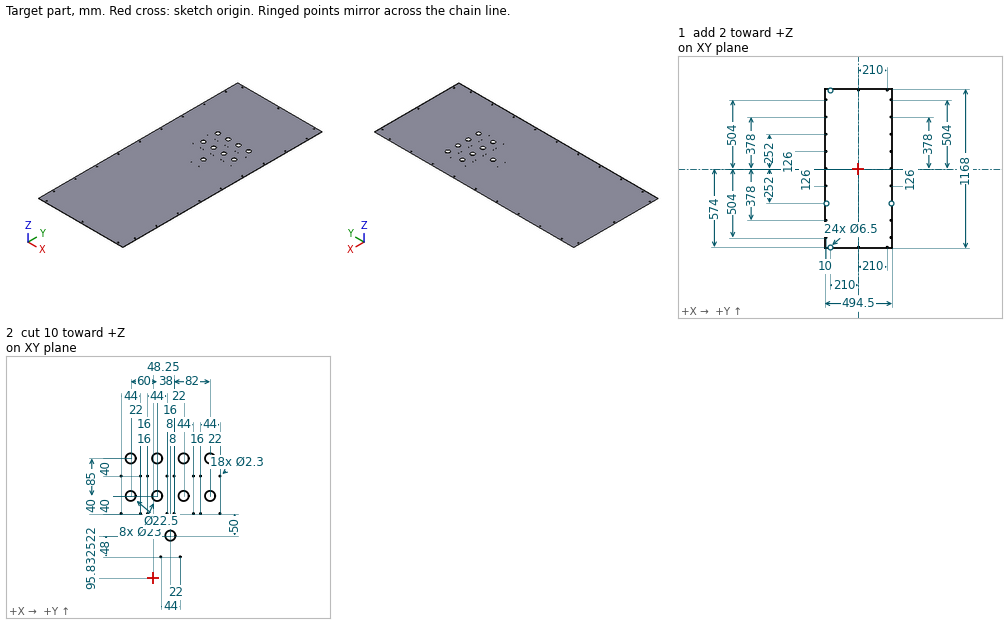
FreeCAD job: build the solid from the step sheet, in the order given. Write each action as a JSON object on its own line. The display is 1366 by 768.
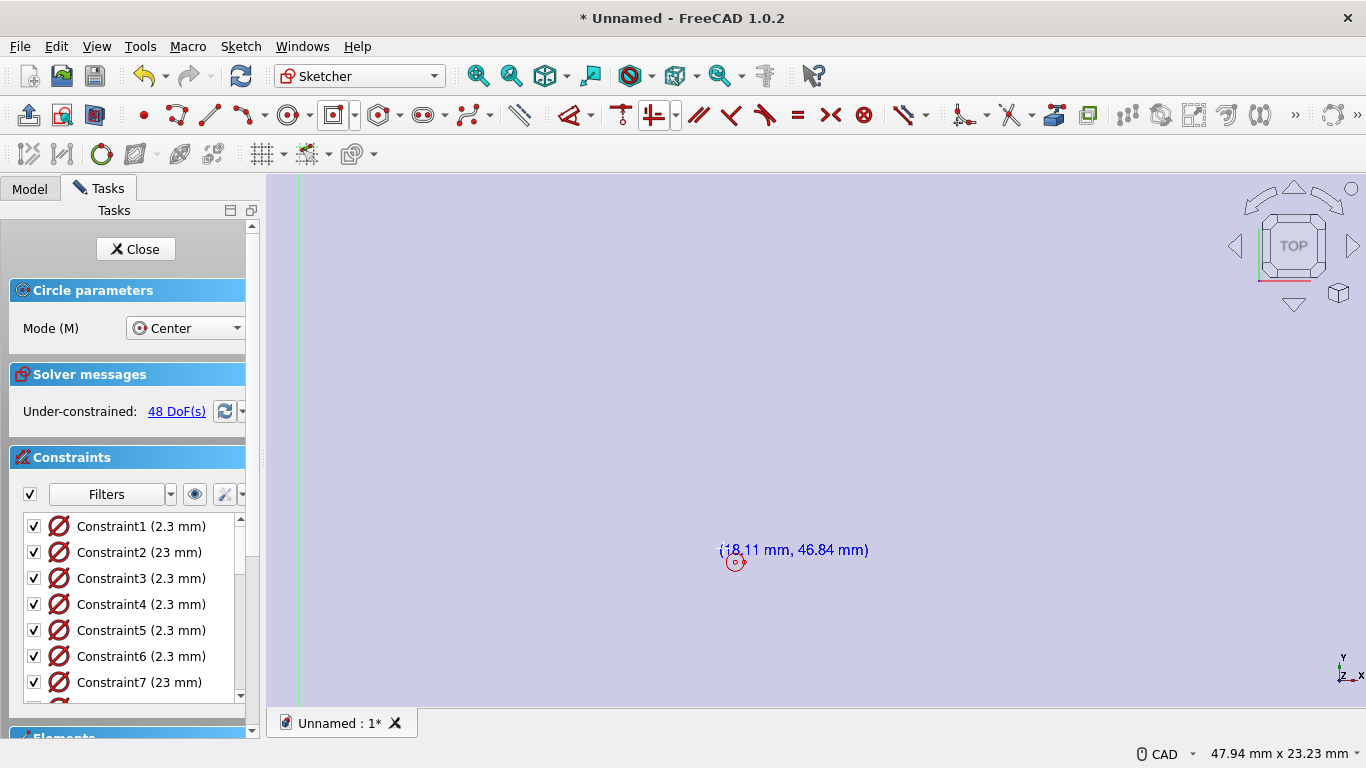
{"action": "scroll", "coordinate": [723, 548], "scroll_direction": "down", "scroll_amount": 15}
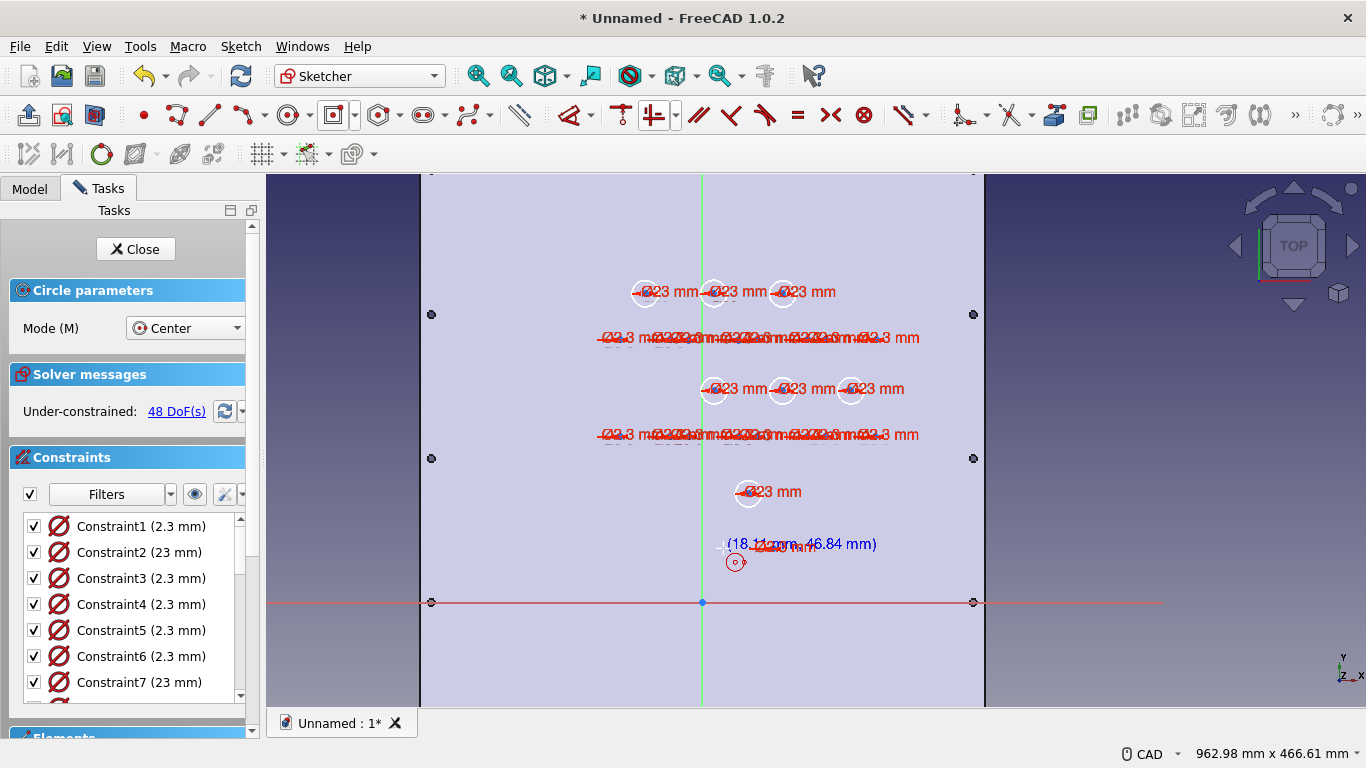
{"action": "left_click", "coordinate": [723, 548]}
{"action": "mouse_move", "coordinate": [724, 547]}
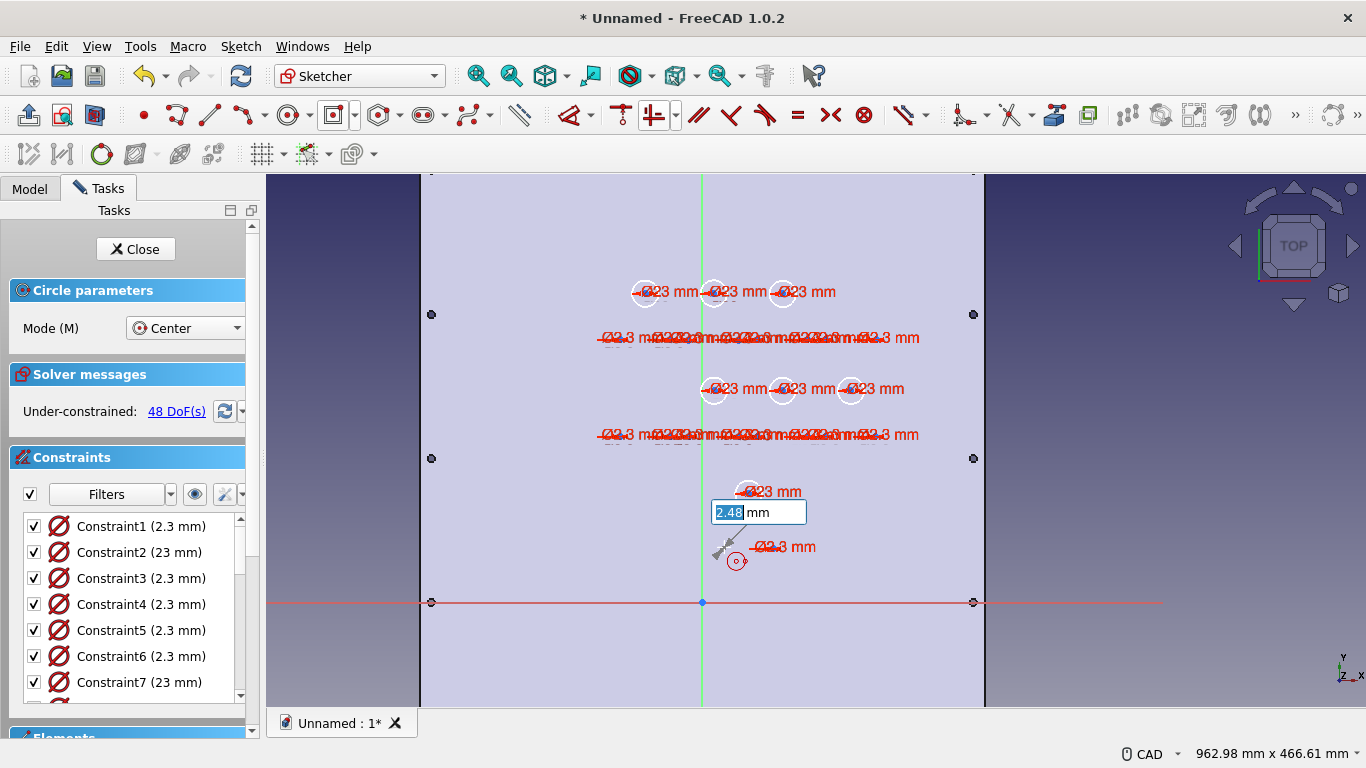
{"action": "type", "text": "2.3"}
{"action": "key", "text": "Return"}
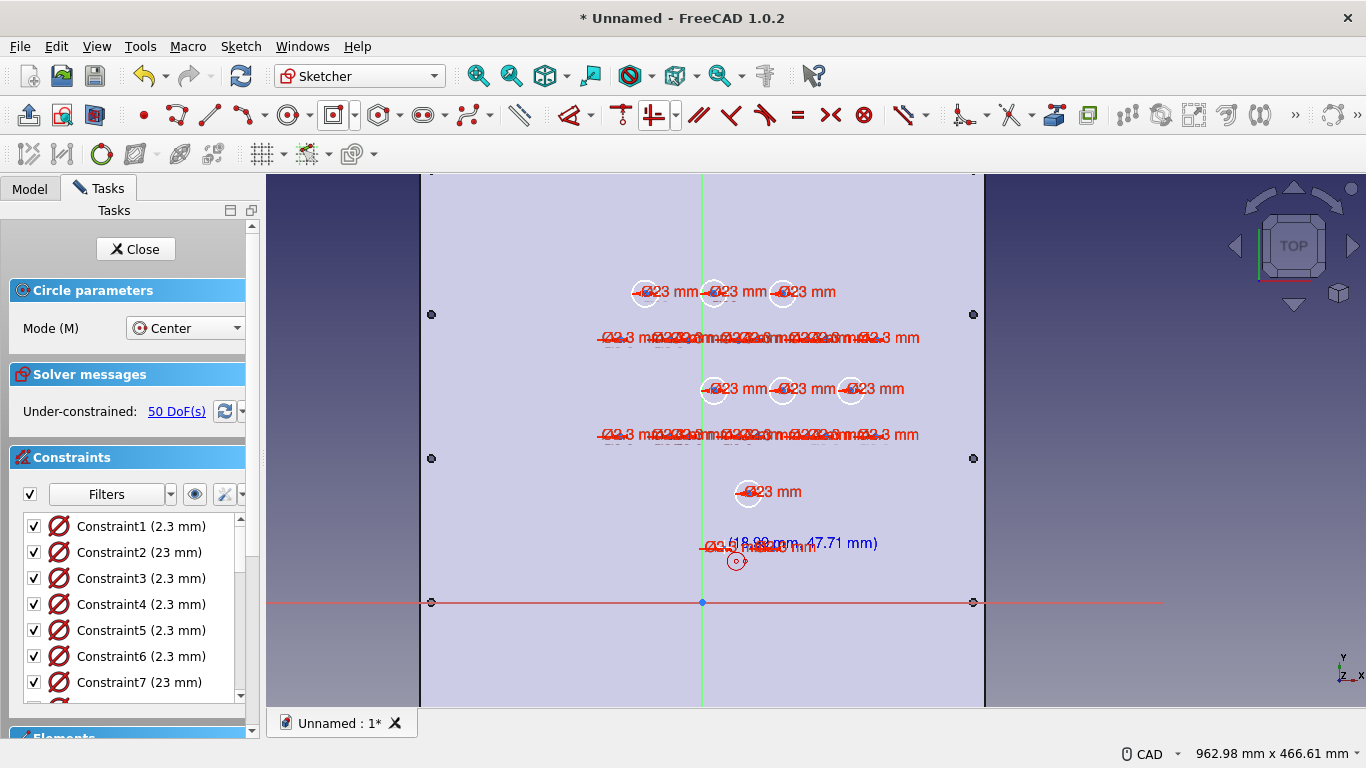
{"action": "scroll", "coordinate": [851, 293], "scroll_direction": "up", "scroll_amount": 3}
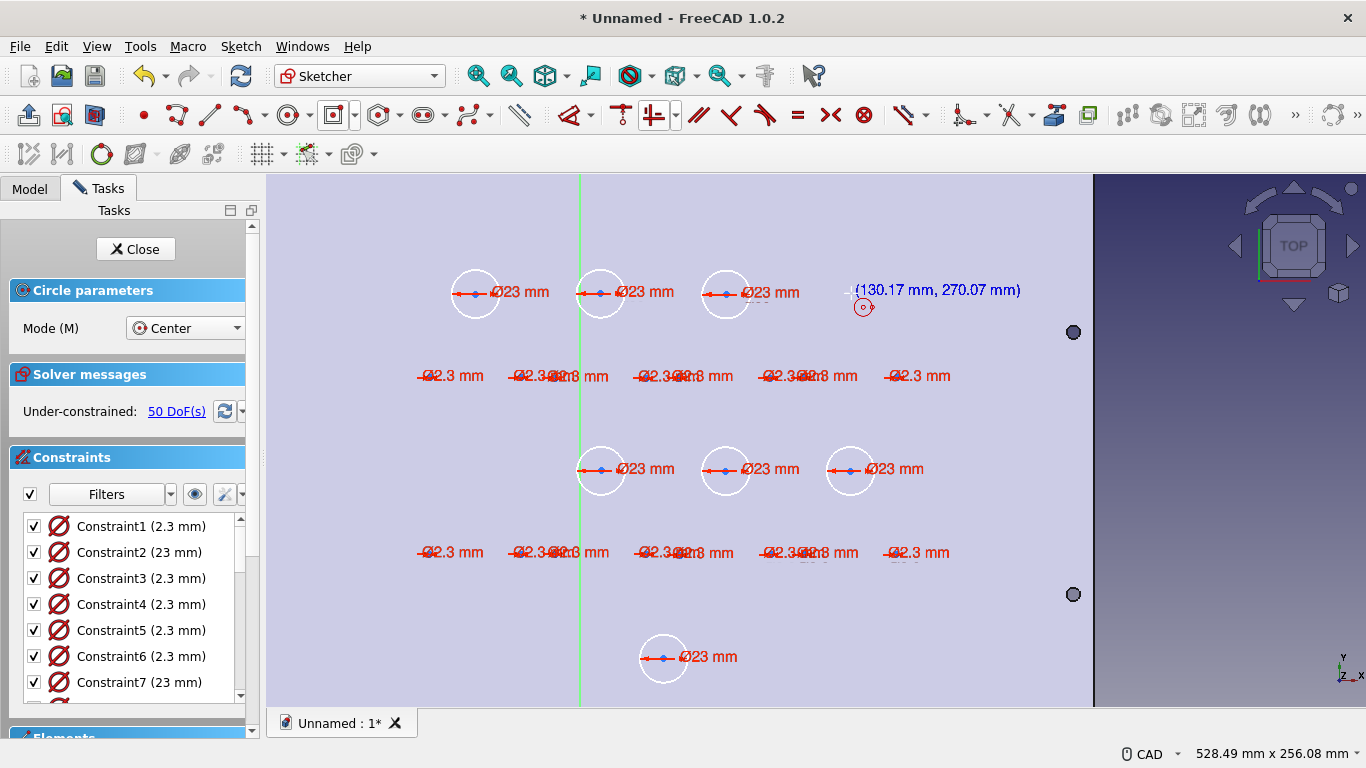
{"action": "left_click", "coordinate": [851, 293]}
{"action": "mouse_move", "coordinate": [868, 276]}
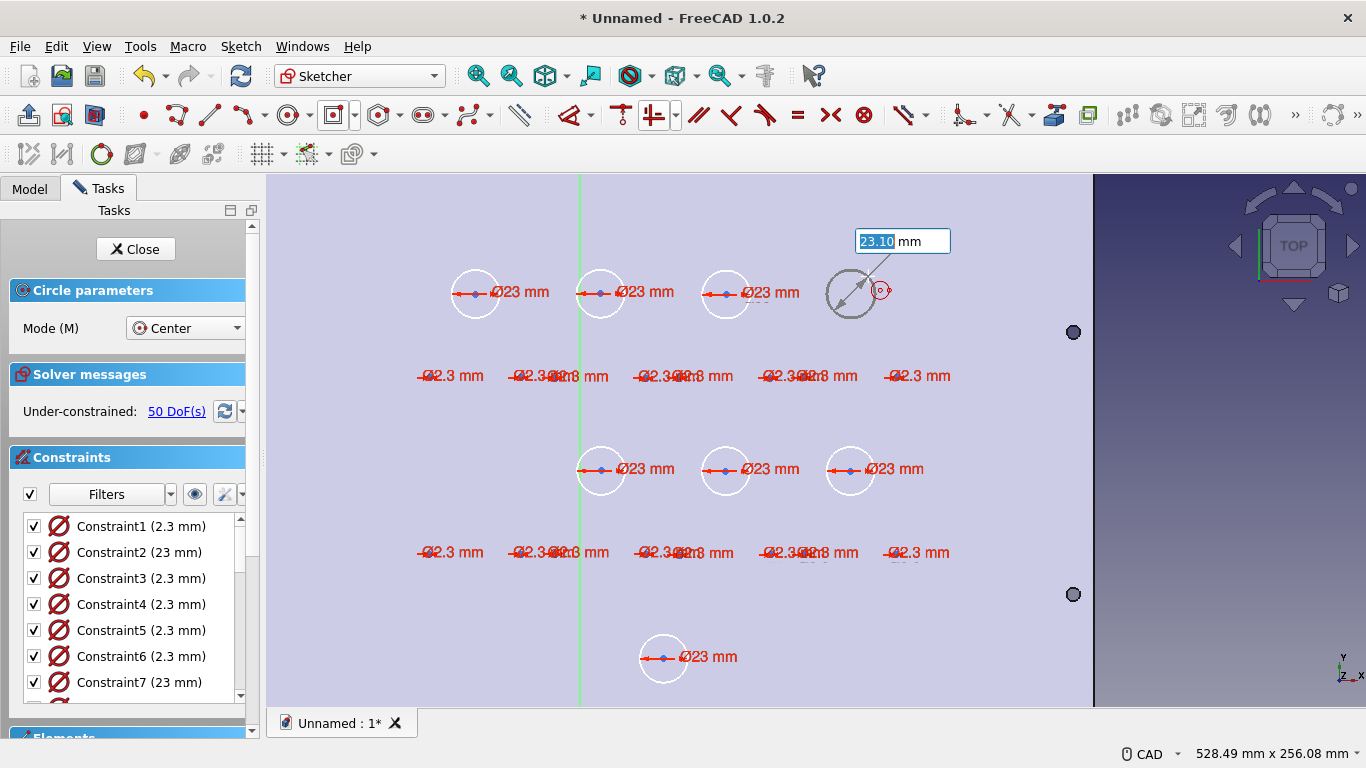
{"action": "type", "text": "23"}
{"action": "key", "text": "Return"}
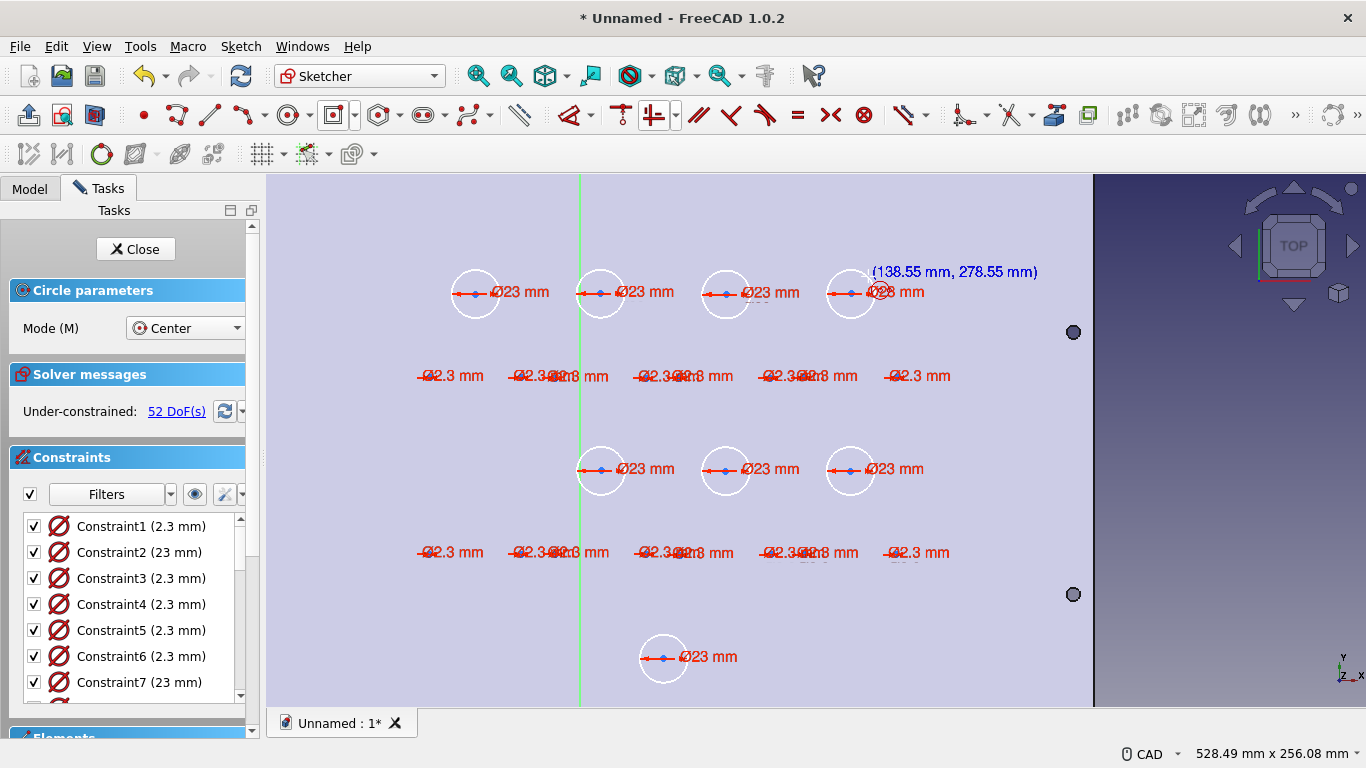
{"action": "left_click", "coordinate": [476, 470]}
{"action": "mouse_move", "coordinate": [493, 453]}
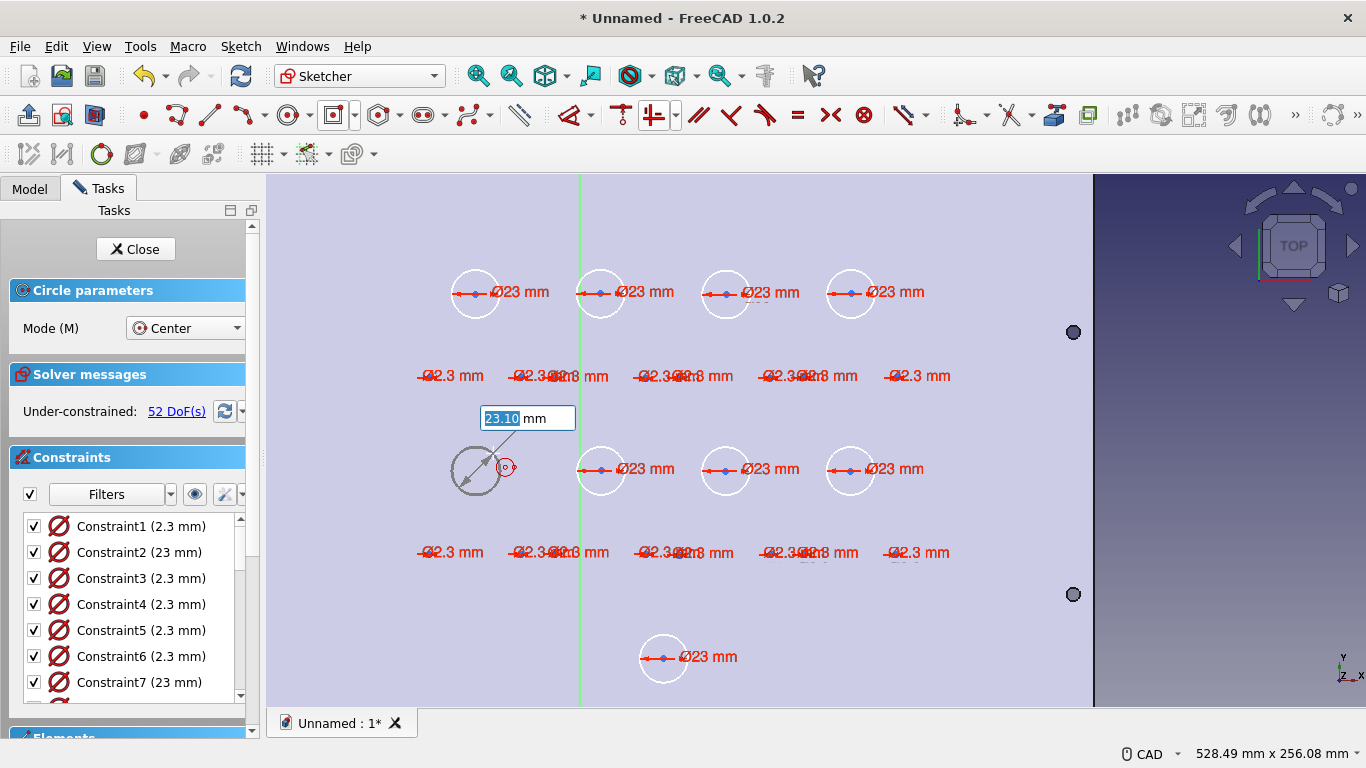
{"action": "type", "text": "22.5"}
{"action": "key", "text": "Return"}
{"action": "key", "text": "Escape"}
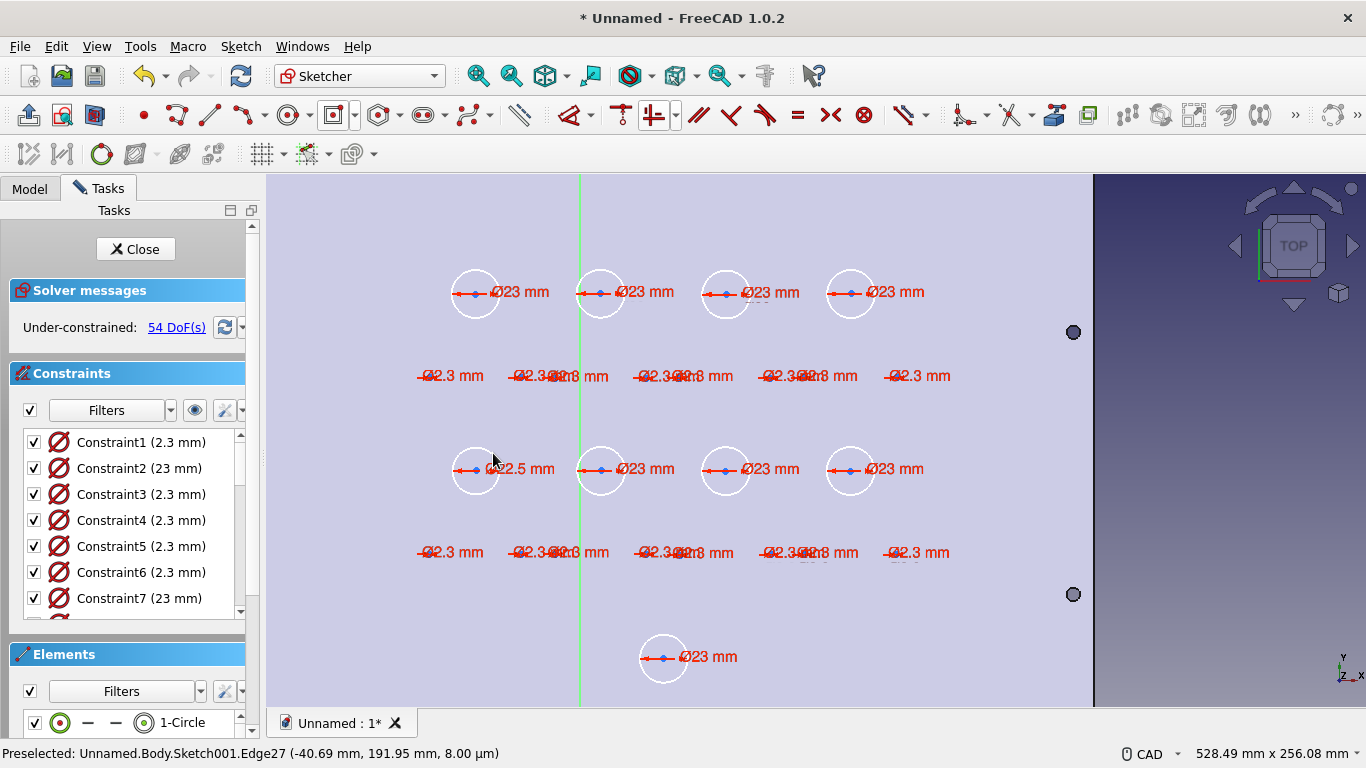
{"action": "left_click", "coordinate": [680, 555]}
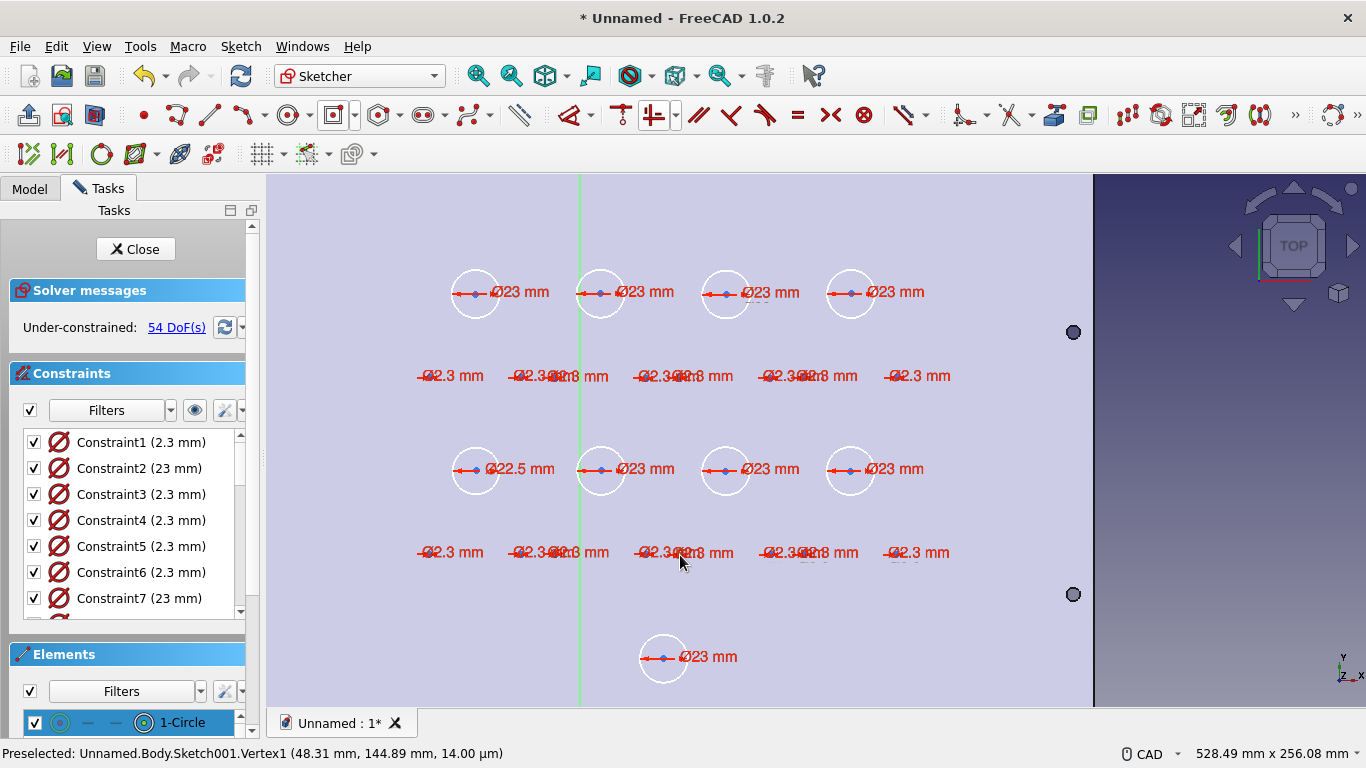
{"action": "left_click", "coordinate": [647, 554]}